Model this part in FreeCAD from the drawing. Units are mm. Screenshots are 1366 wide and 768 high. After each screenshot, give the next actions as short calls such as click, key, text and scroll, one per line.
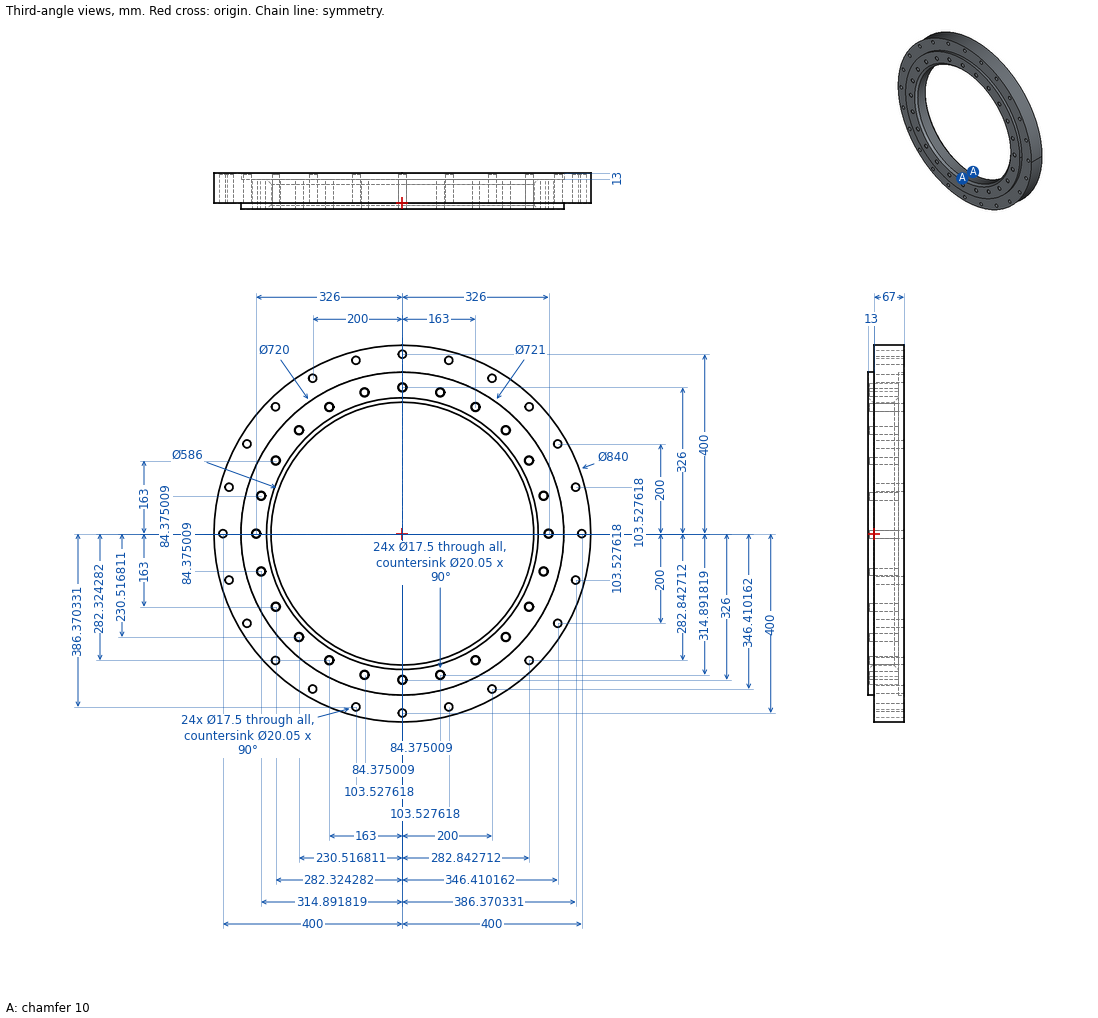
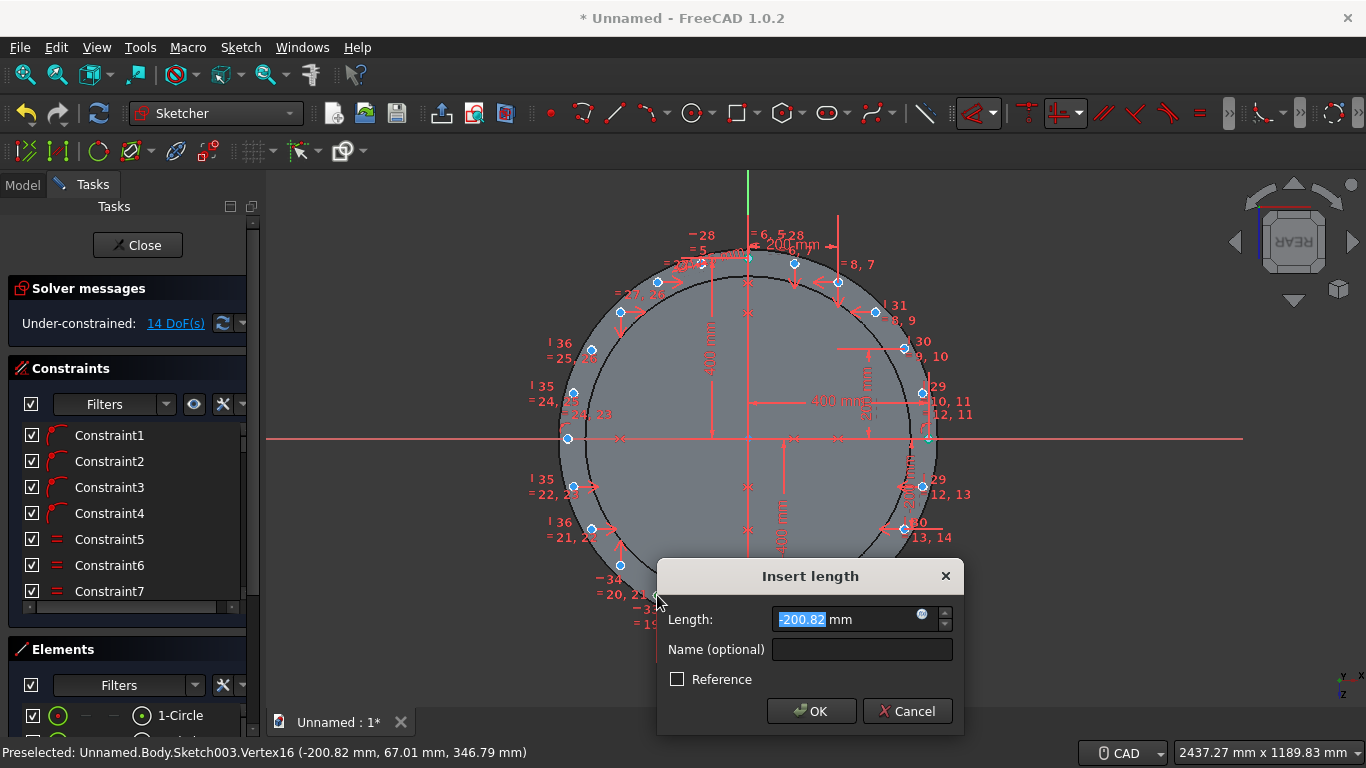
text(-200)
key(Return)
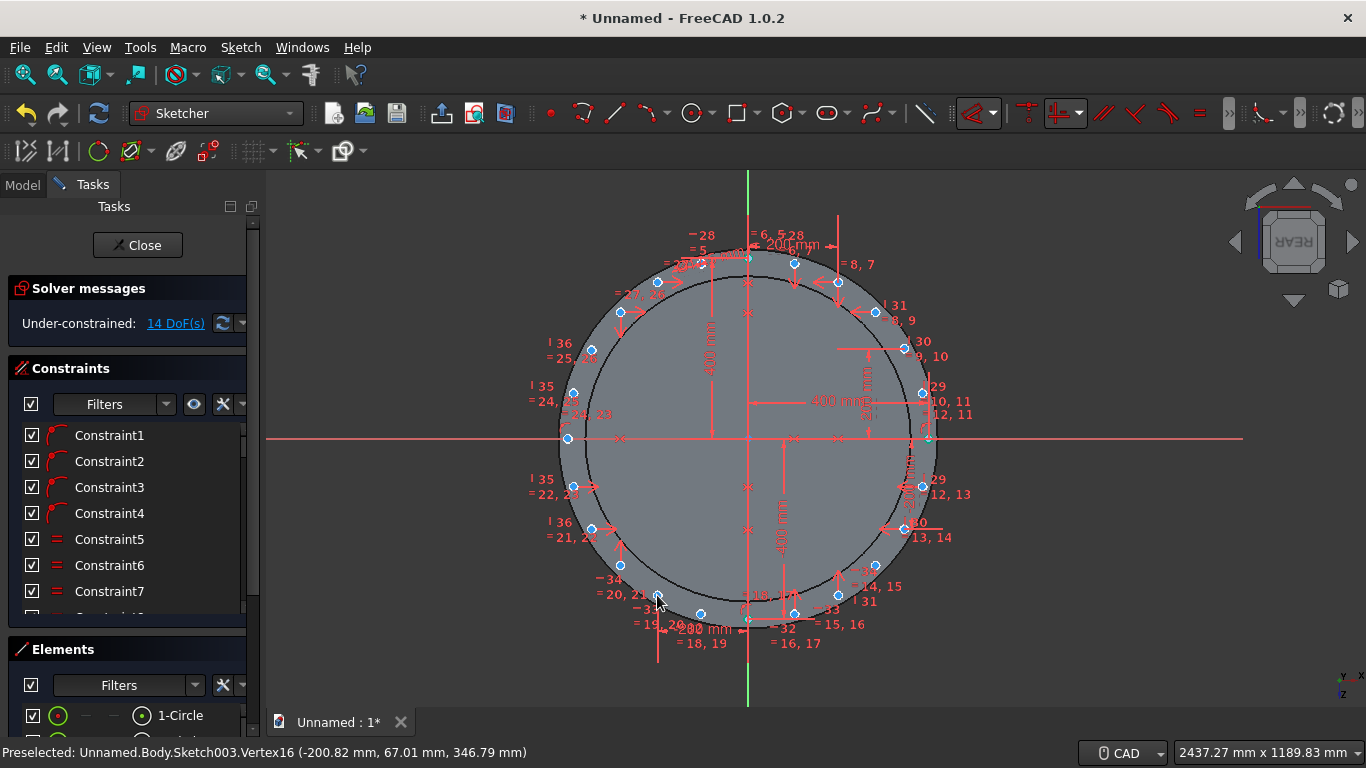
click(568, 439)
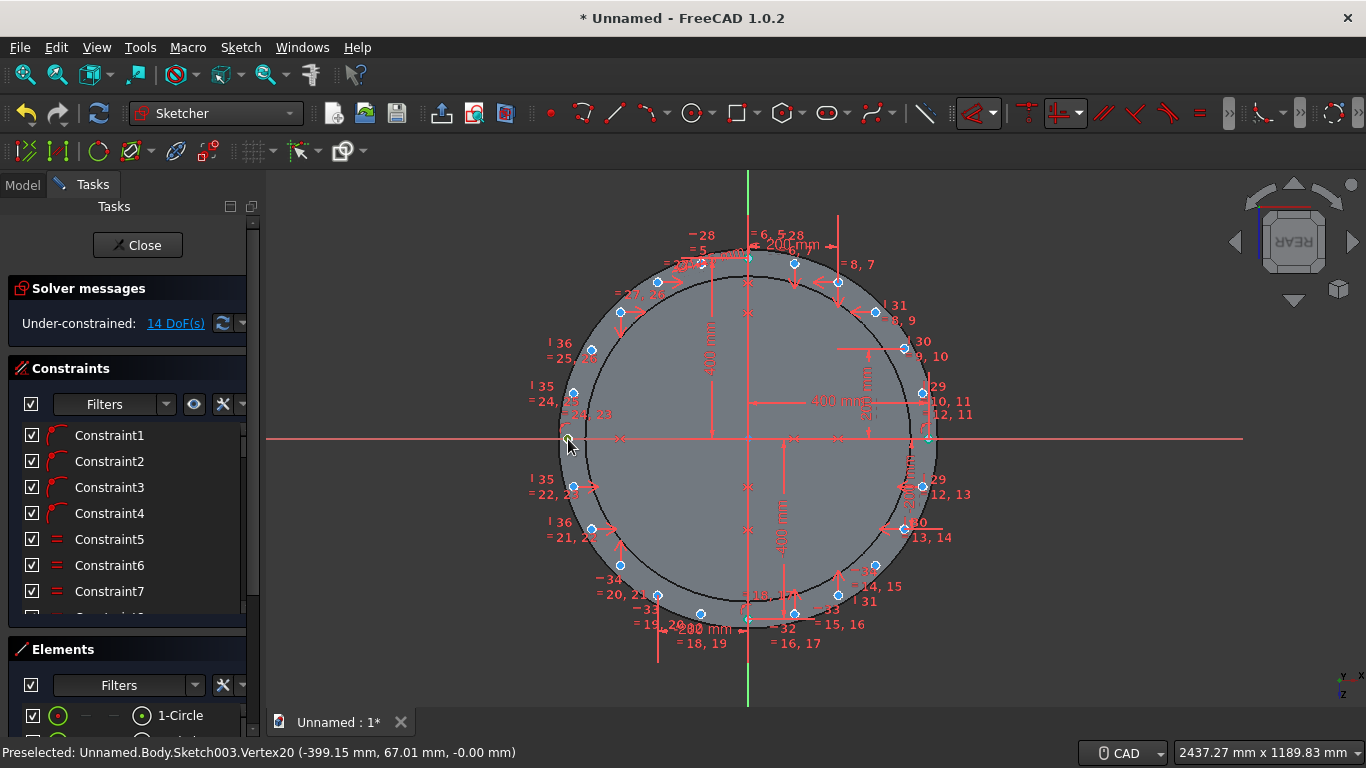
key(l)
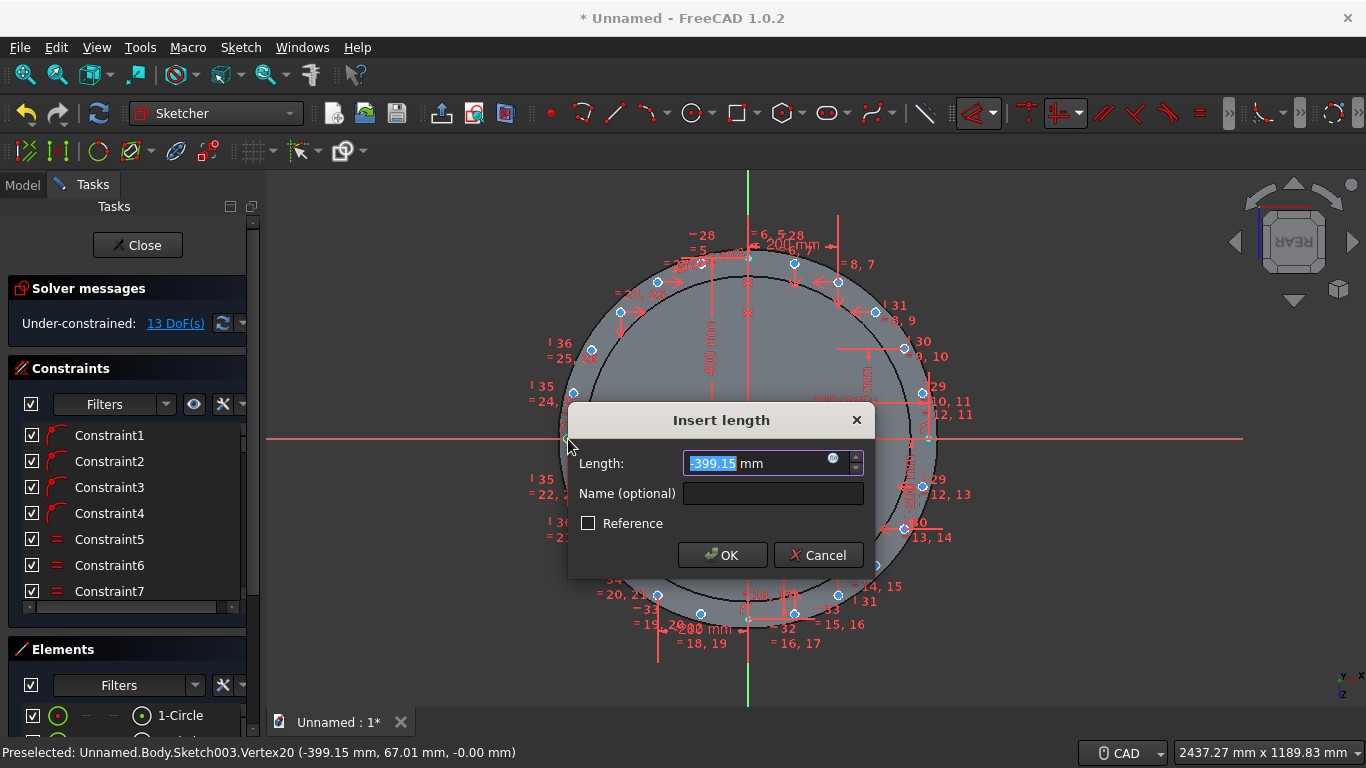
text(-400)
key(Return)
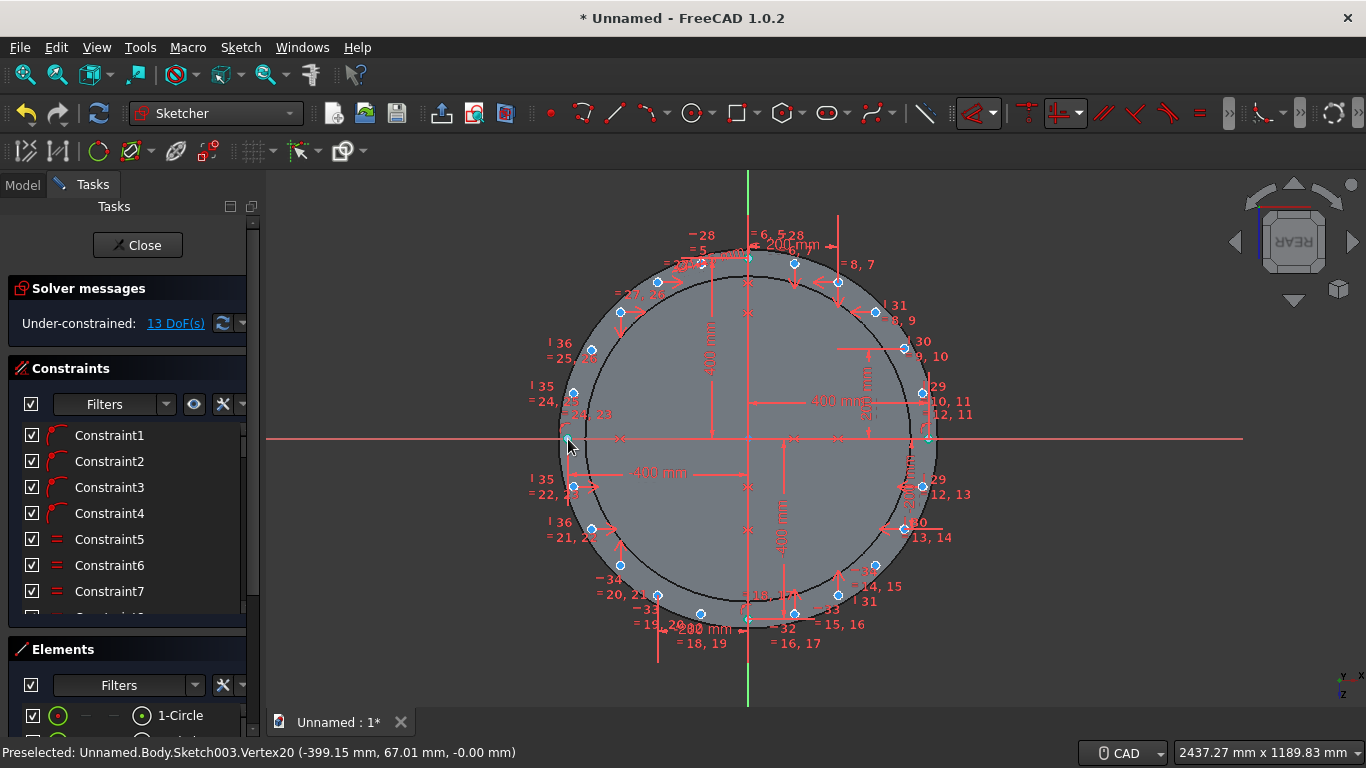
scroll(592, 350, up, 4)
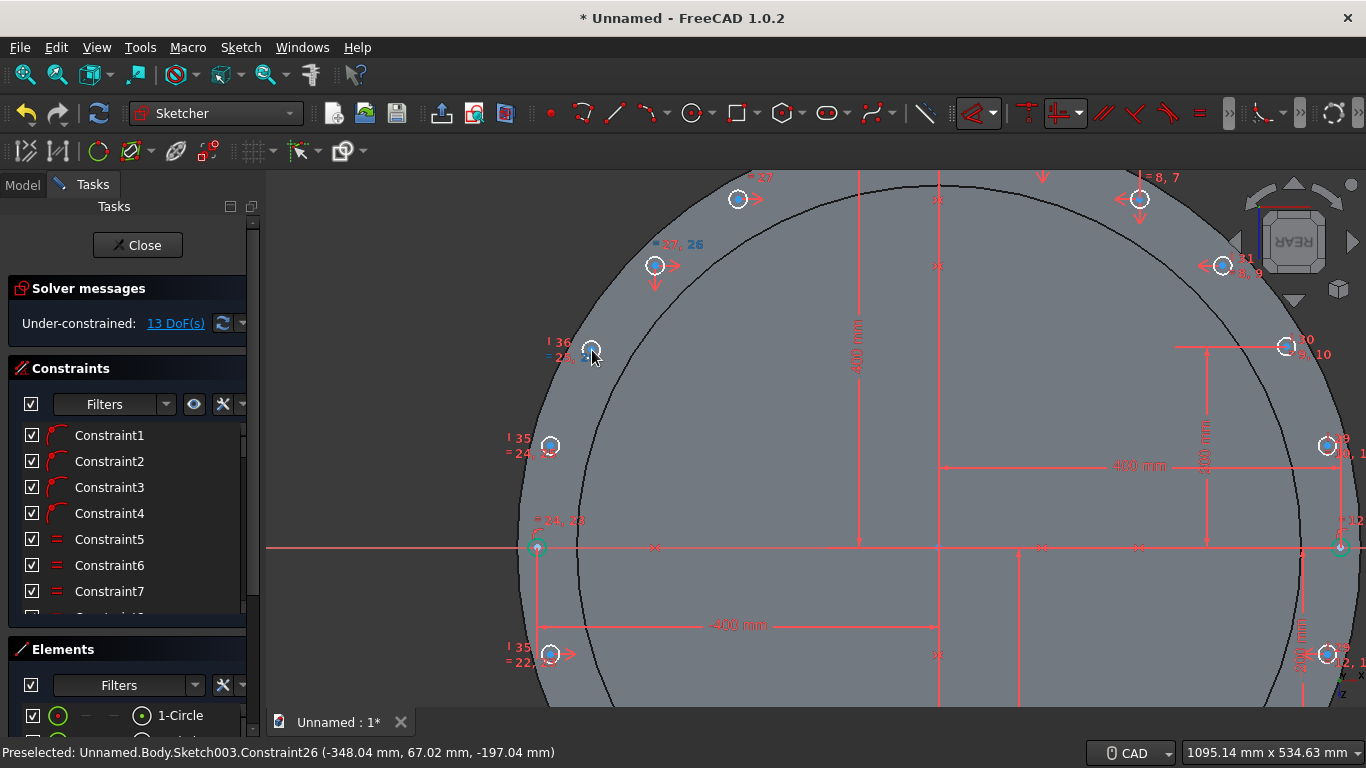
scroll(591, 350, up, 4)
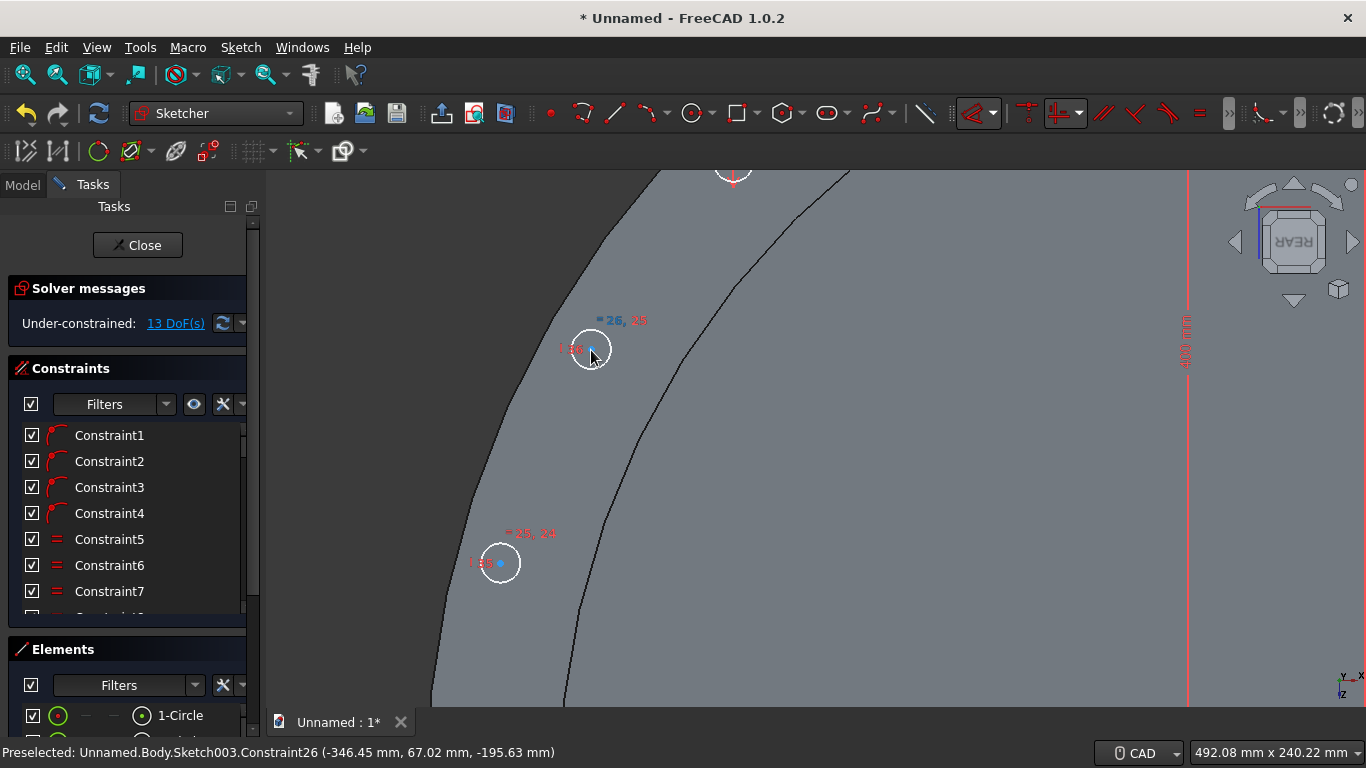
click(591, 349)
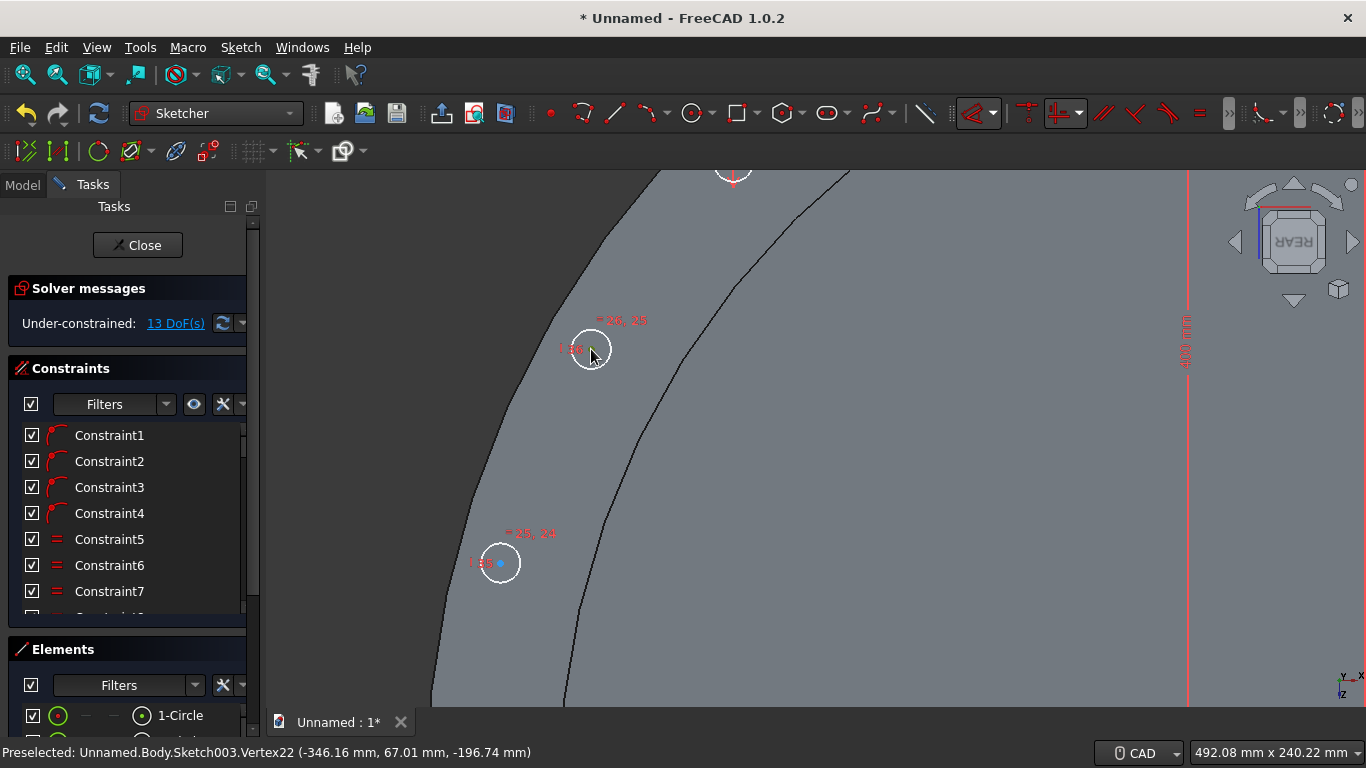
click(996, 114)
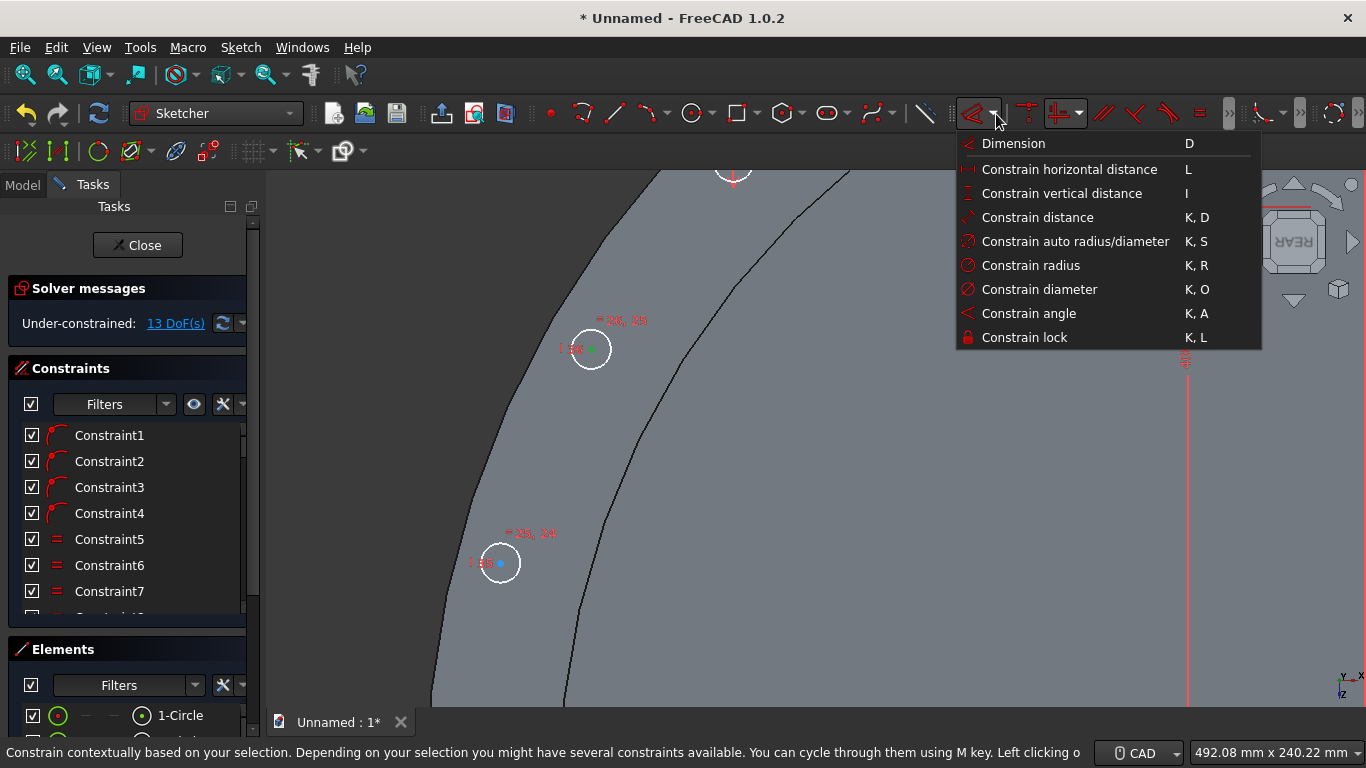
click(1109, 193)